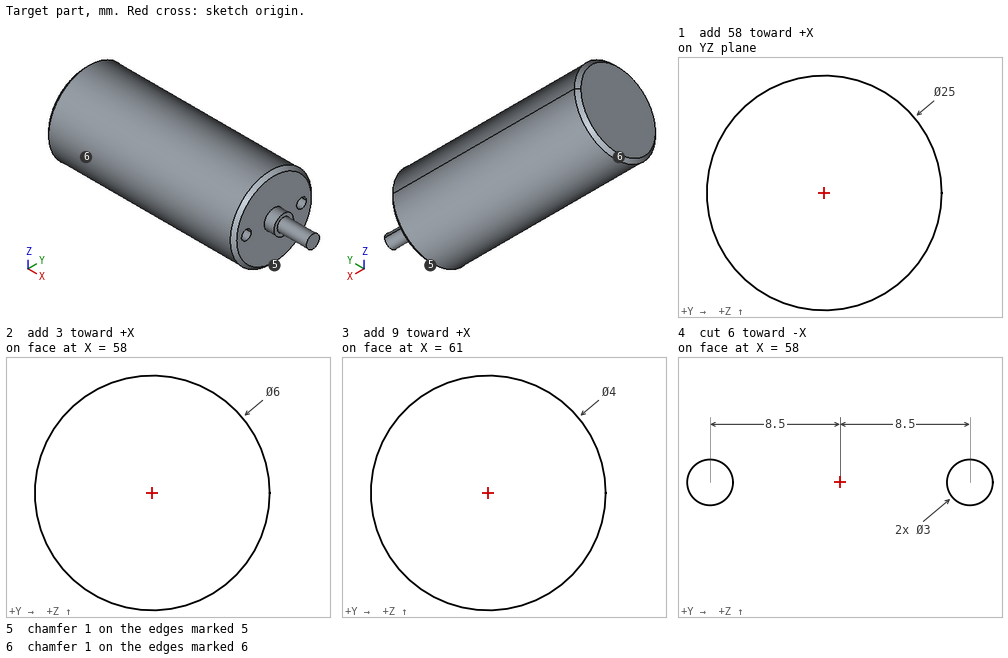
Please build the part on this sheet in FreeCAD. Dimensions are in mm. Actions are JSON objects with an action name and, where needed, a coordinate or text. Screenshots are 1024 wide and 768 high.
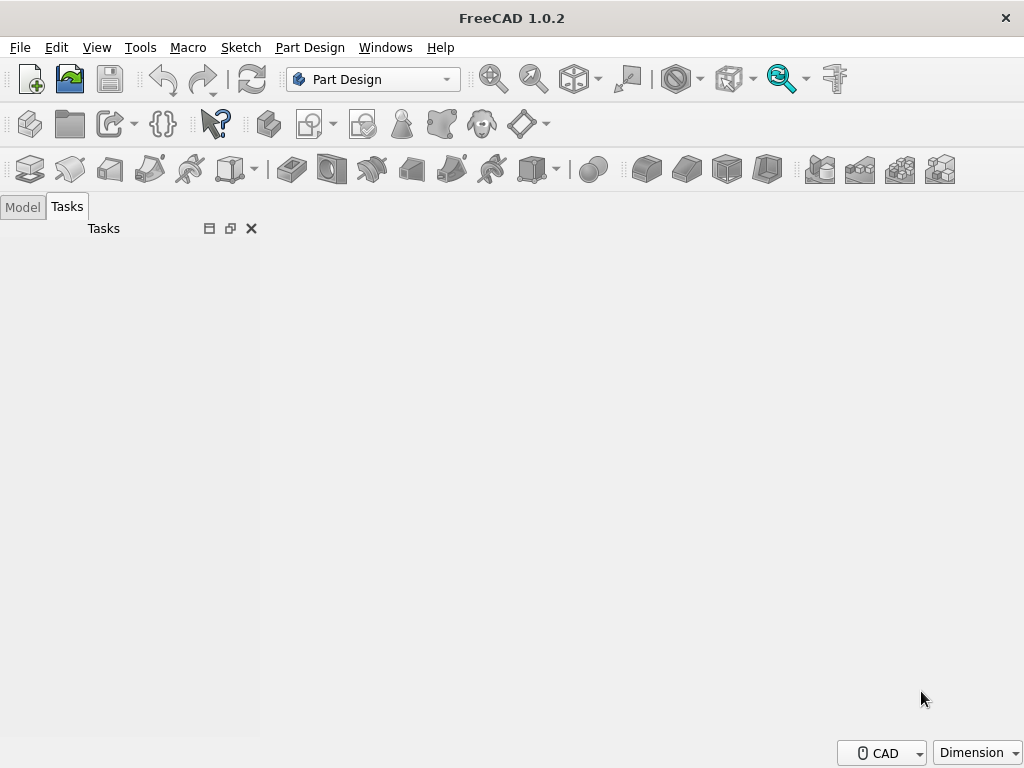
{"action": "left_click", "coordinate": [30, 80]}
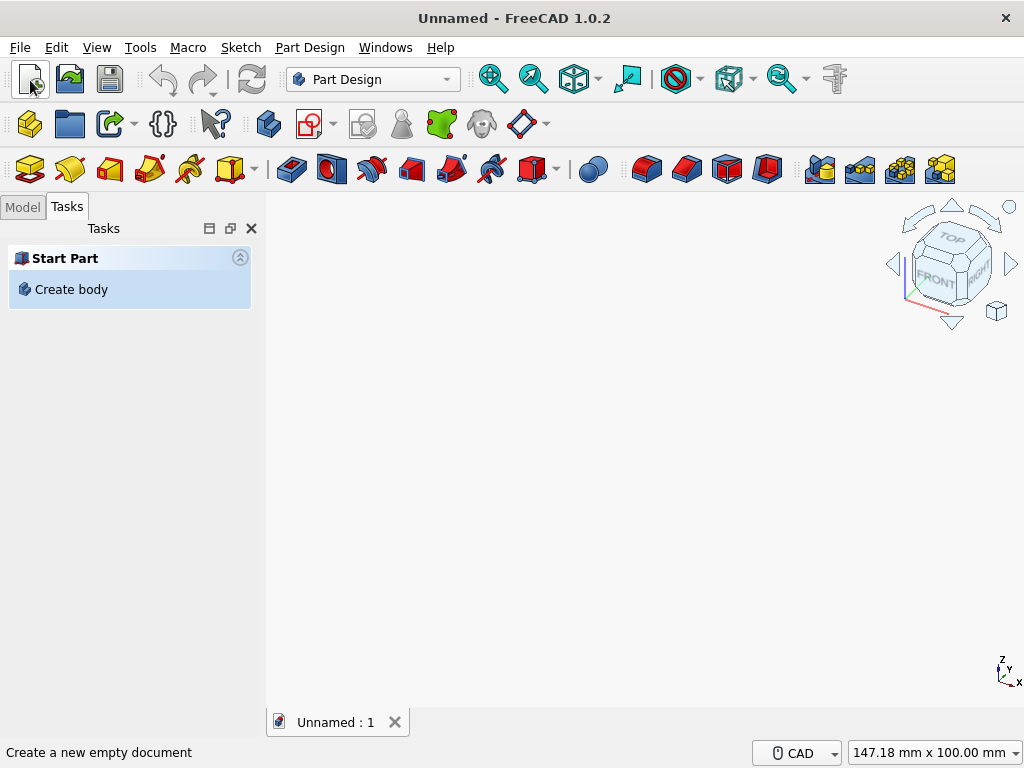
{"action": "left_click", "coordinate": [310, 124]}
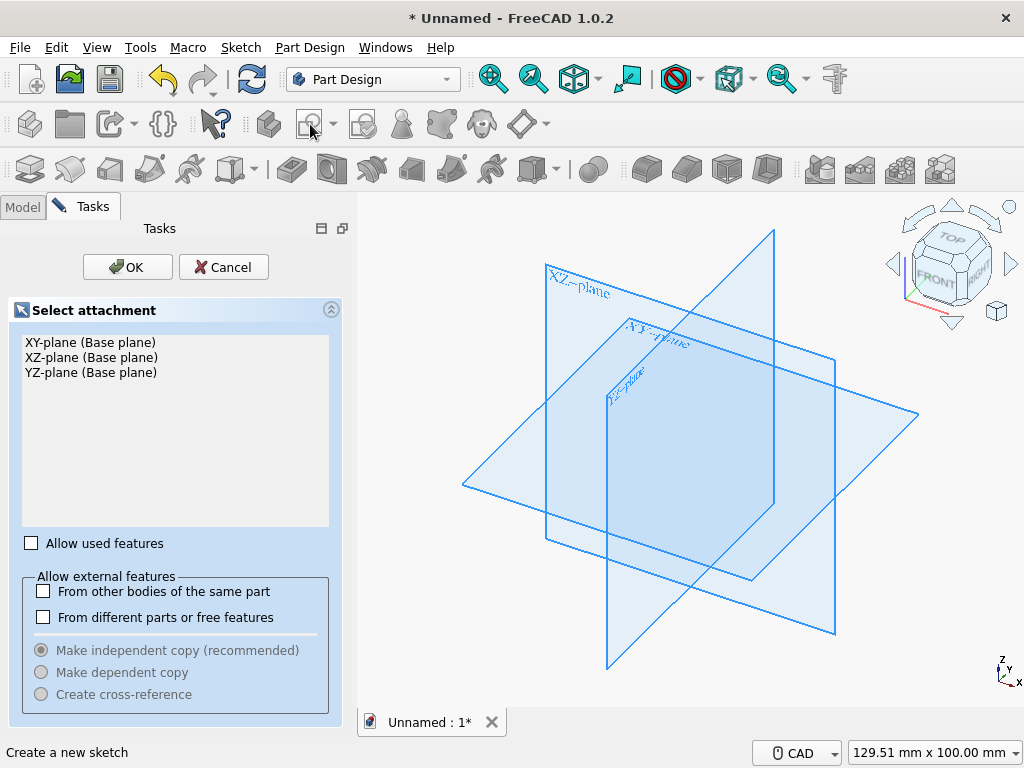
{"action": "left_click", "coordinate": [82, 372]}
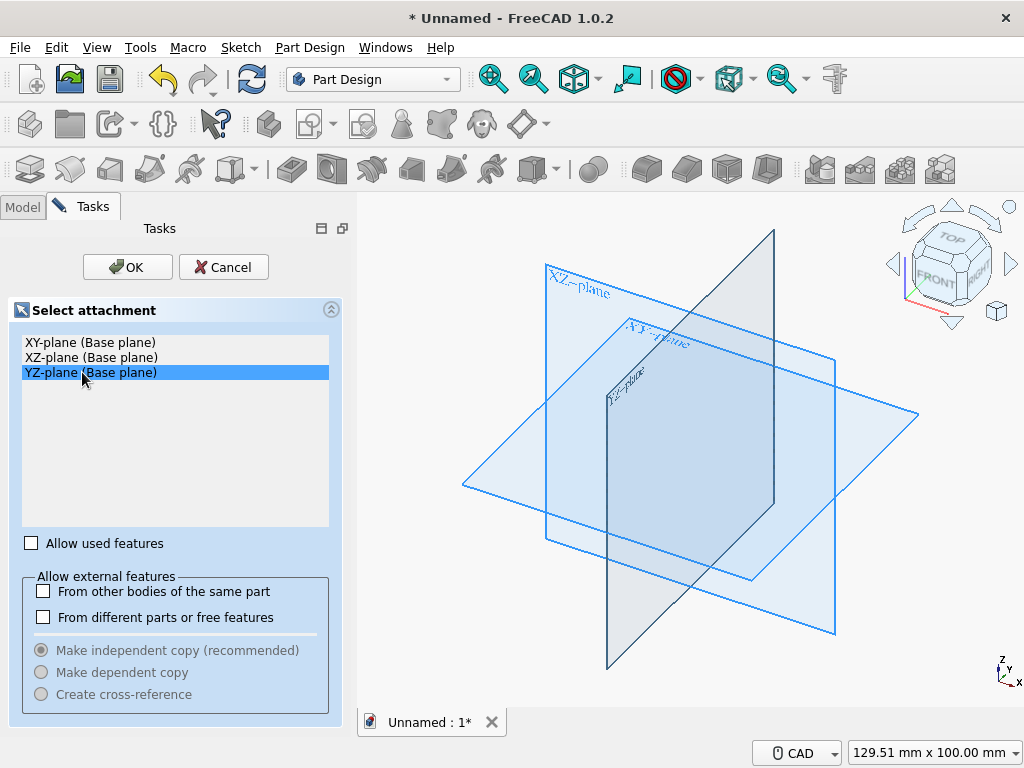
{"action": "left_click", "coordinate": [128, 267]}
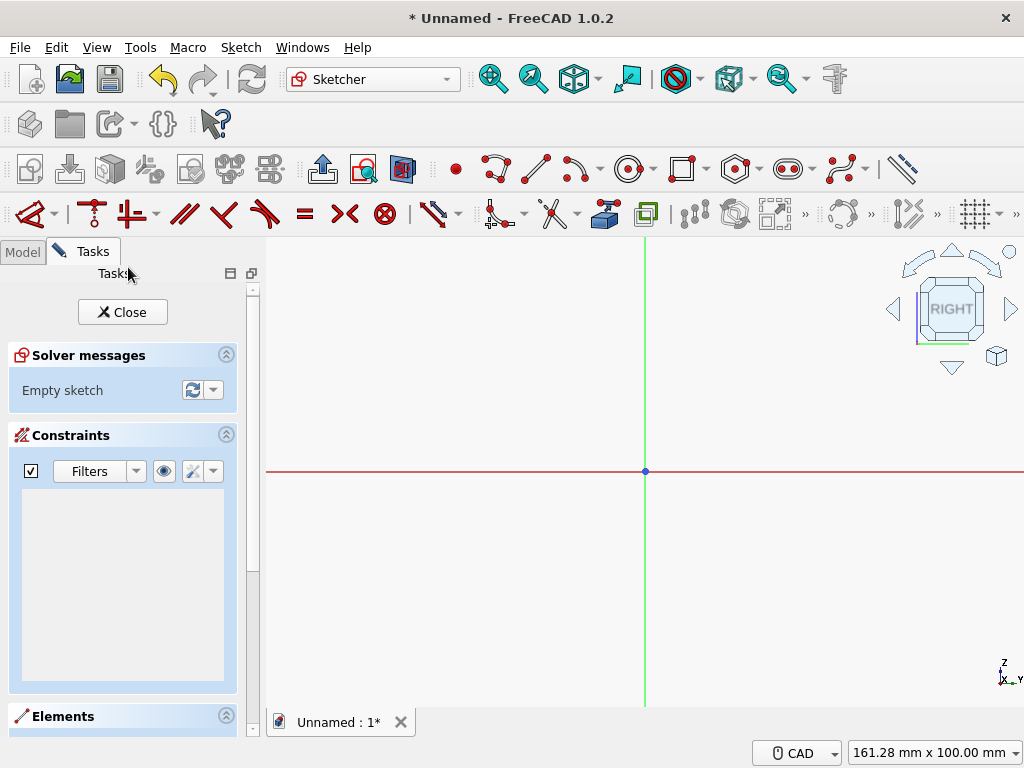
{"action": "scroll", "coordinate": [685, 472], "scroll_direction": "up", "scroll_amount": 5}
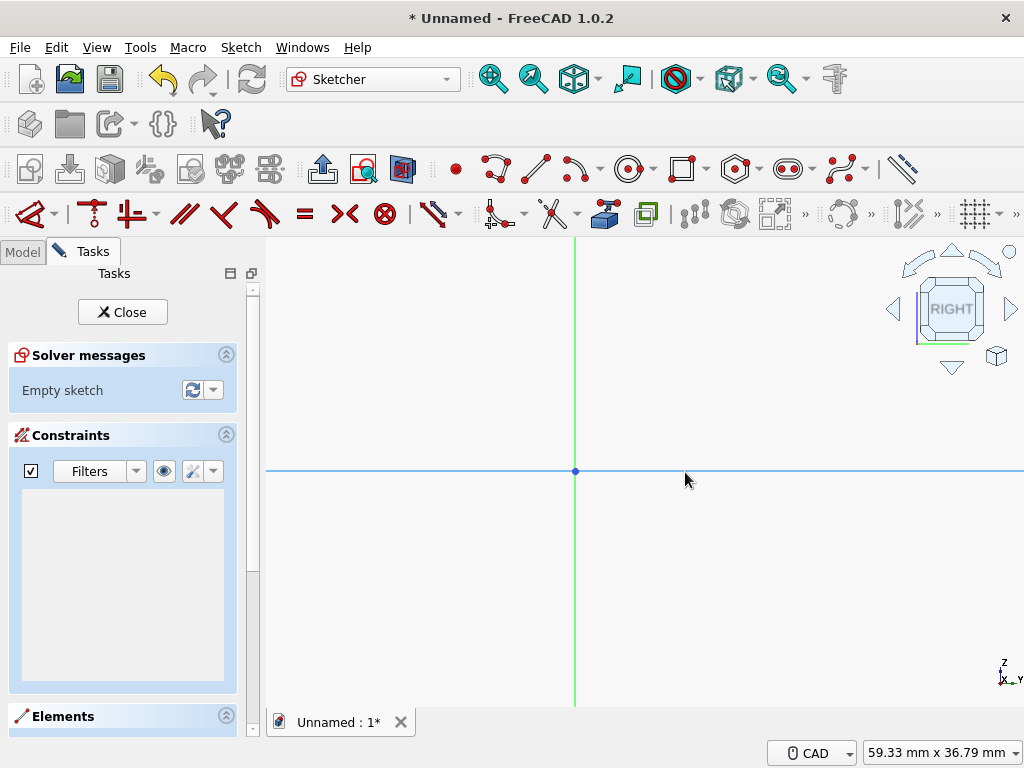
{"action": "key", "text": "g c"}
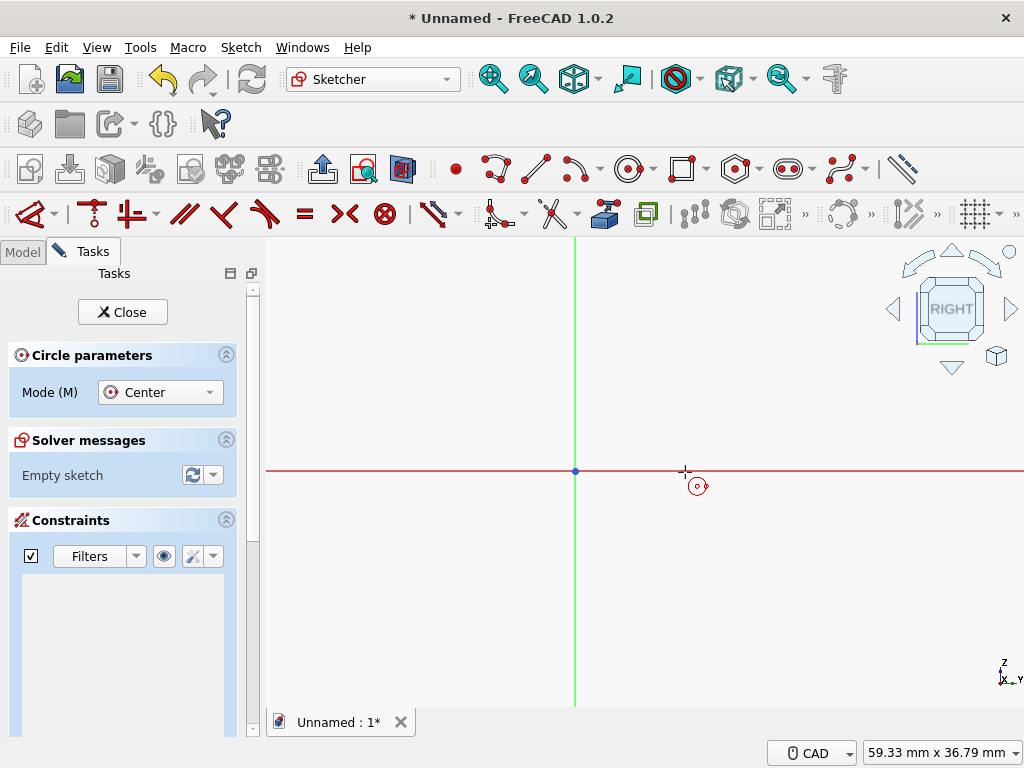
{"action": "left_click", "coordinate": [575, 471]}
{"action": "left_click", "coordinate": [688, 358]}
{"action": "key", "text": "Escape"}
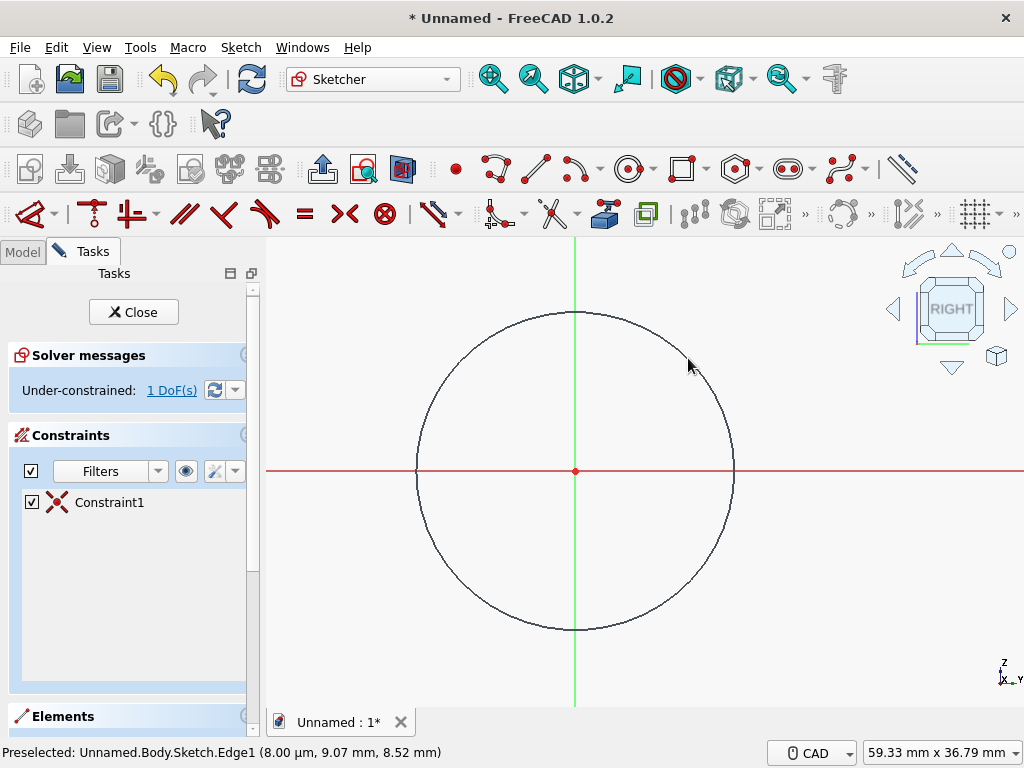
{"action": "left_click", "coordinate": [30, 214]}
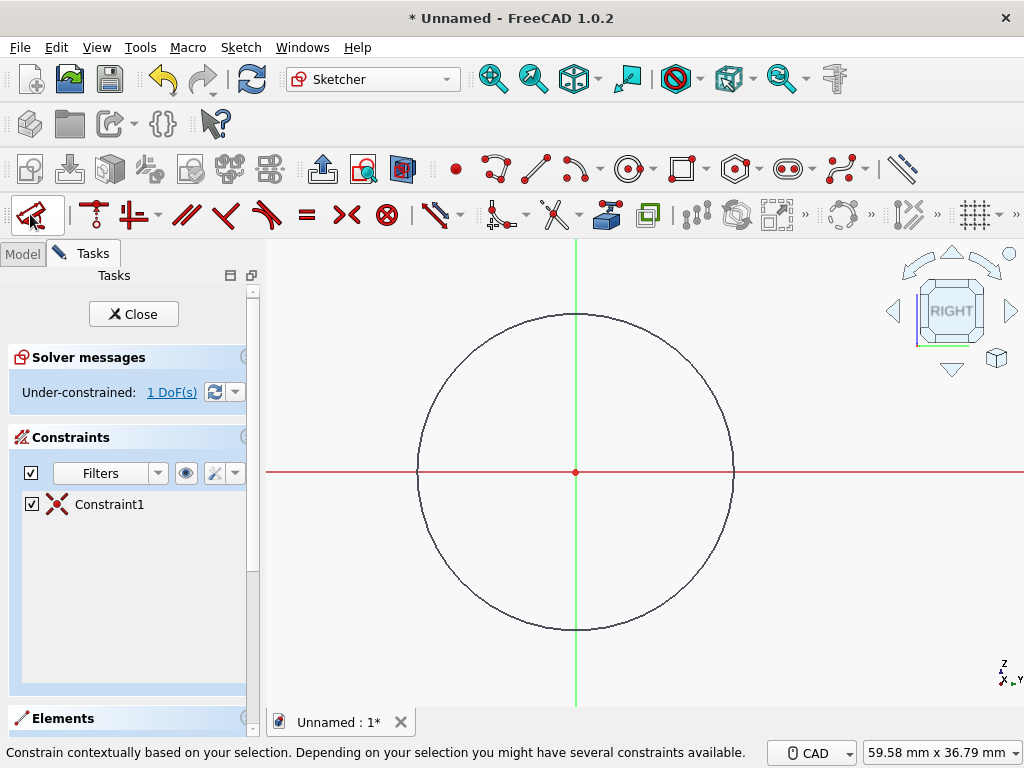
{"action": "left_click", "coordinate": [687, 360]}
{"action": "left_click", "coordinate": [710, 337]}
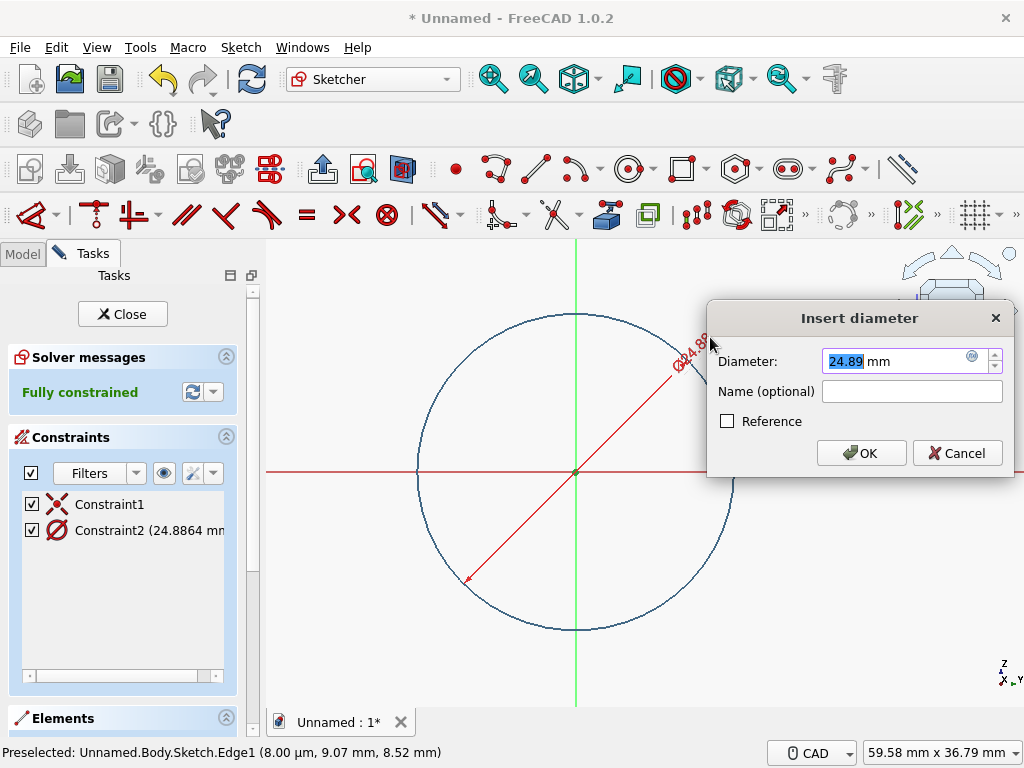
{"action": "type", "text": "25"}
{"action": "key", "text": "Return"}
{"action": "key", "text": "Escape"}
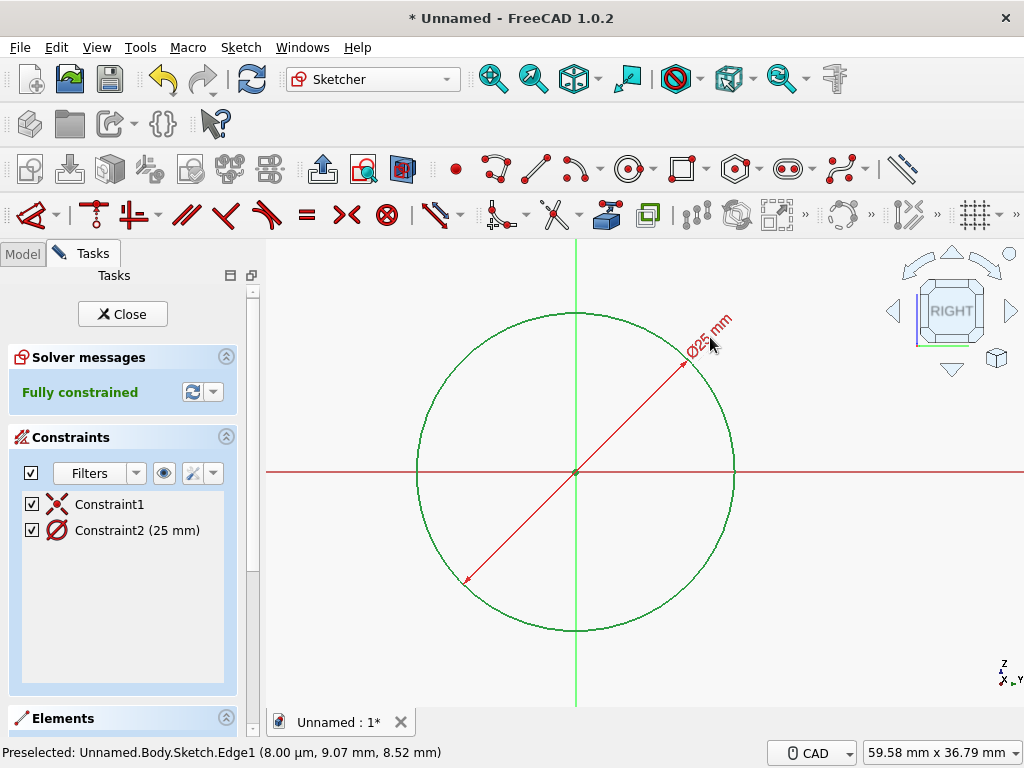
{"action": "left_click", "coordinate": [123, 314]}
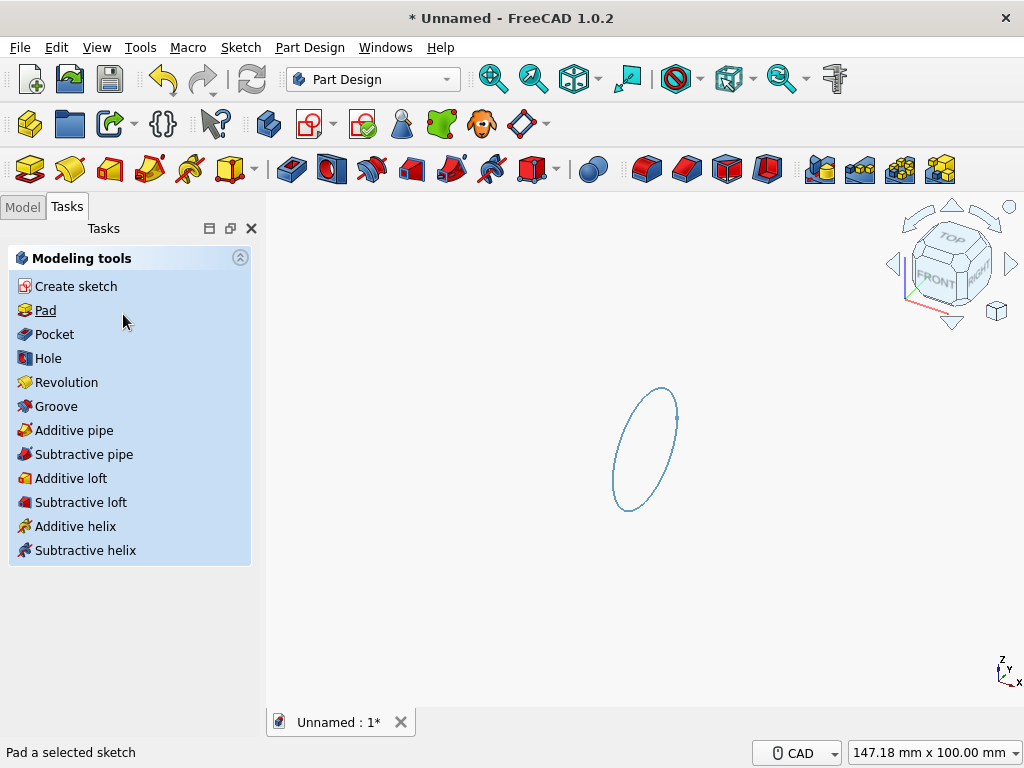
{"action": "left_click", "coordinate": [30, 170]}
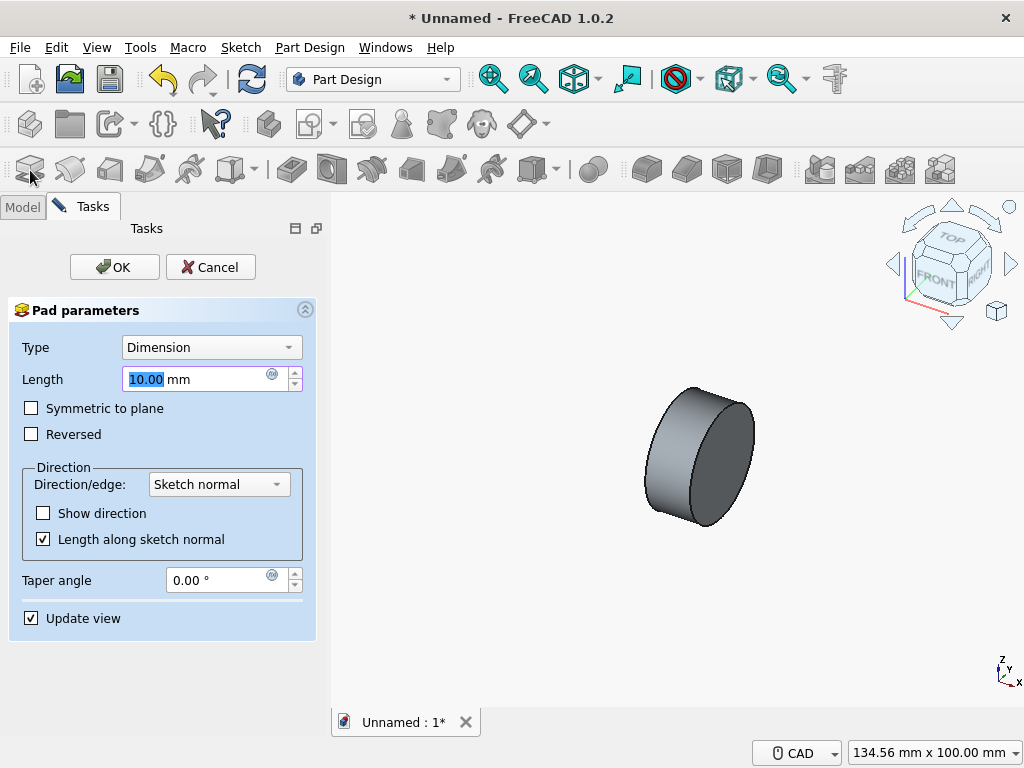
{"action": "type", "text": "58"}
{"action": "key", "text": "Tab"}